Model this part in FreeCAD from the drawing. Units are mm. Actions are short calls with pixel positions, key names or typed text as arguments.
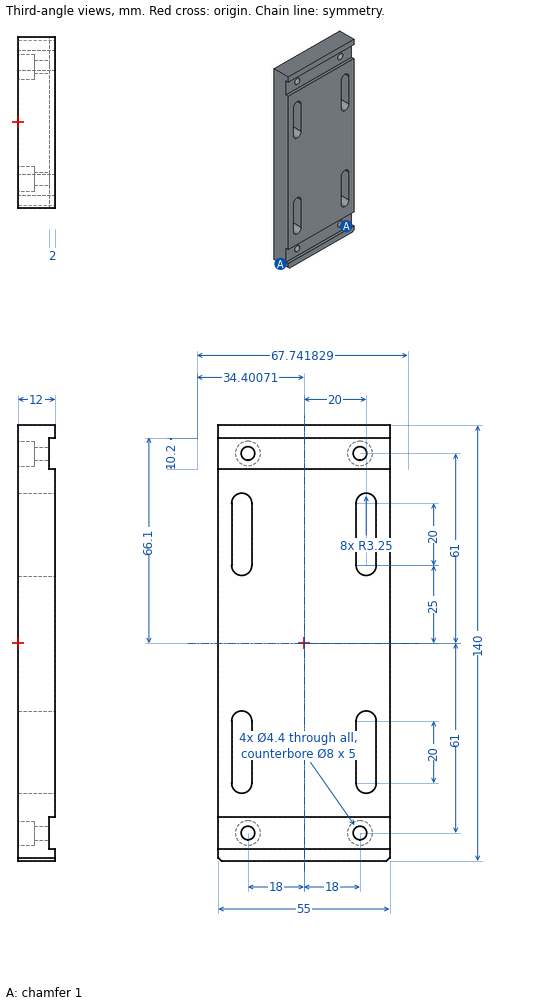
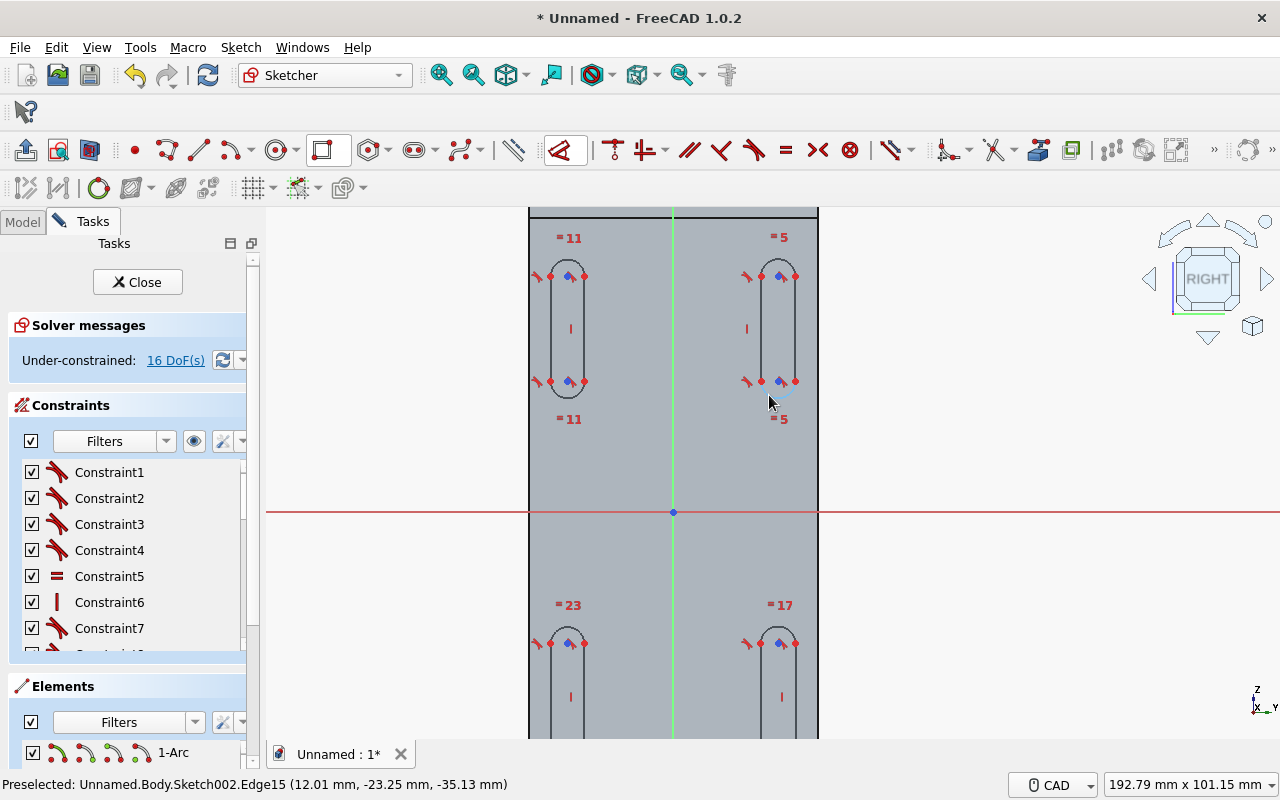
click(768, 395)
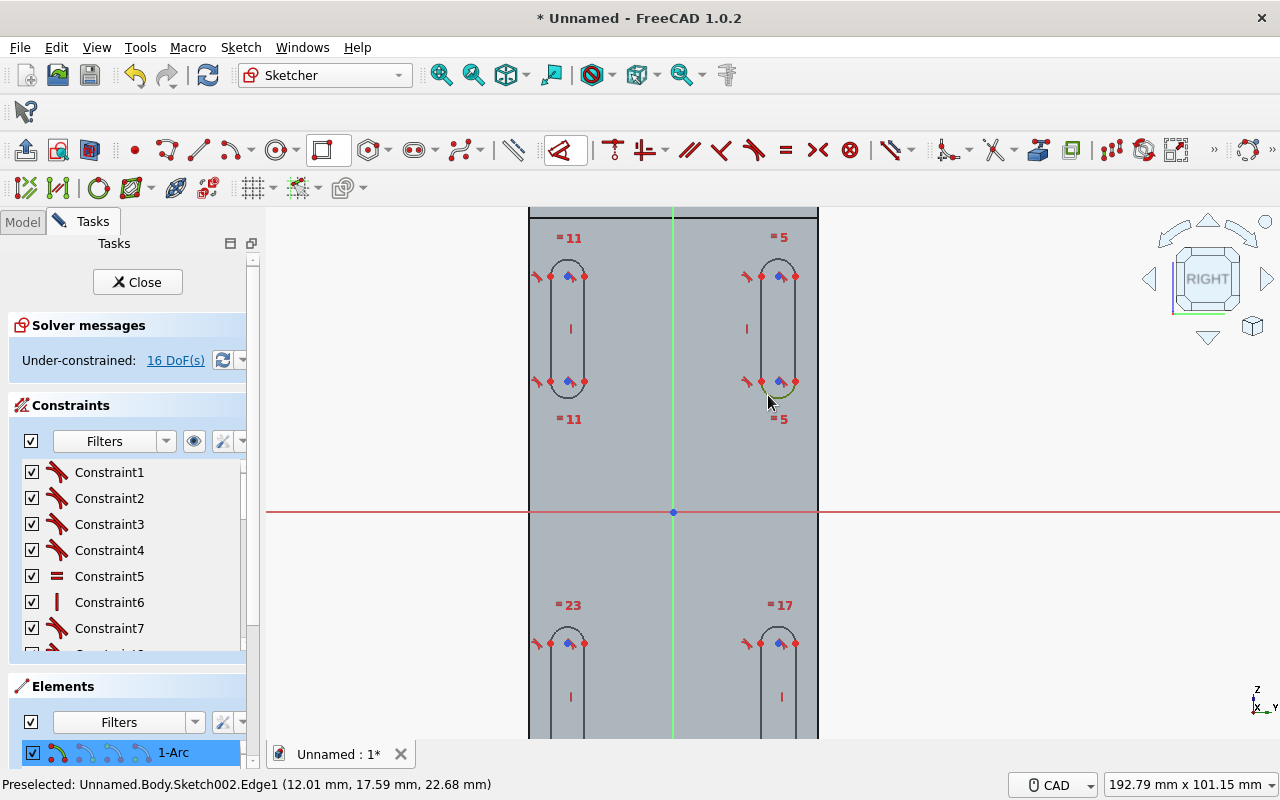
click(558, 395)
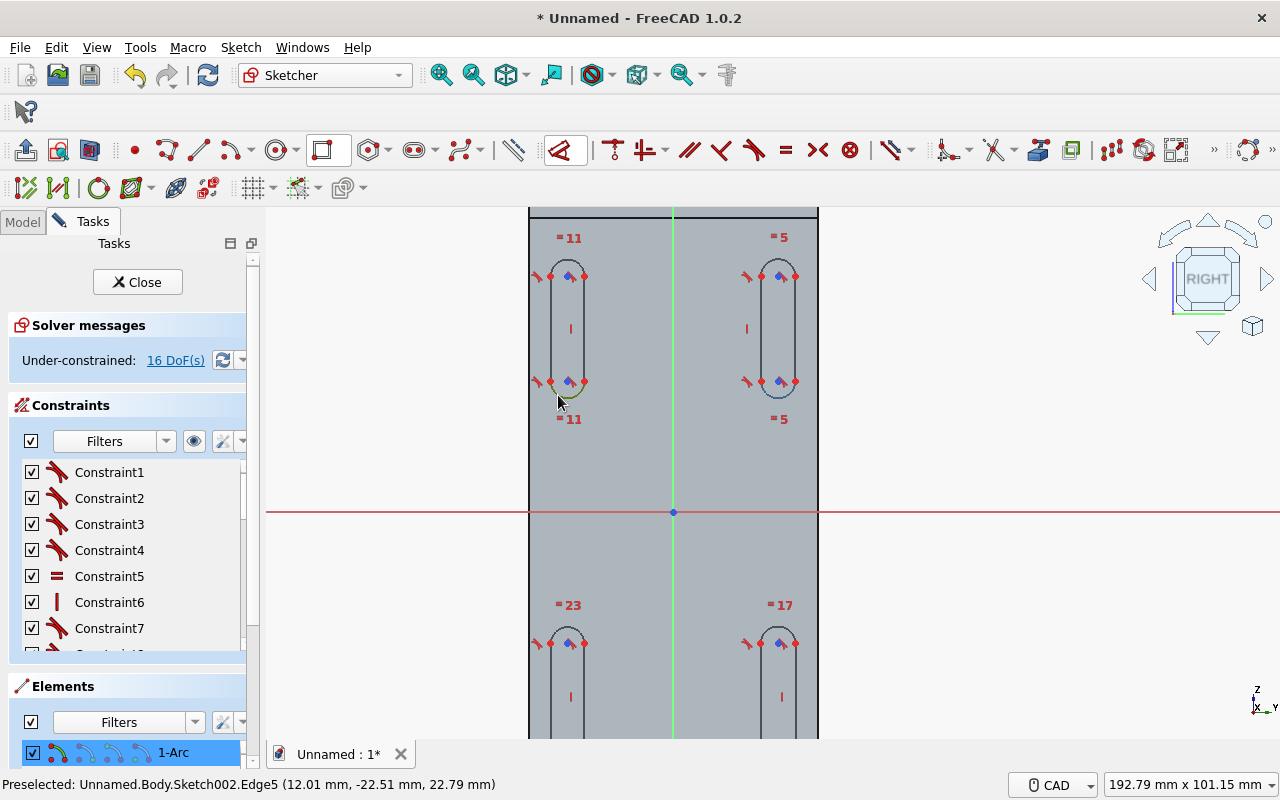
scroll(768, 393, down, 2)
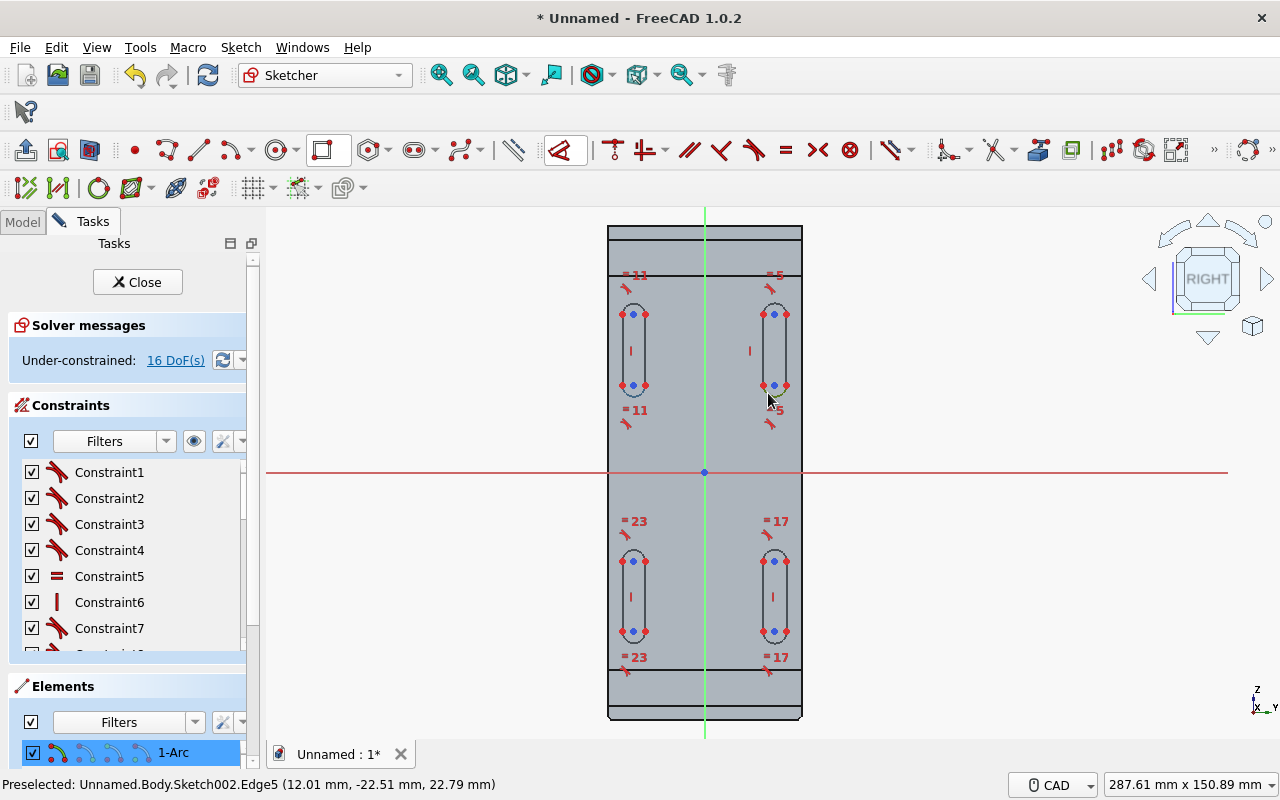
scroll(768, 641, up, 2)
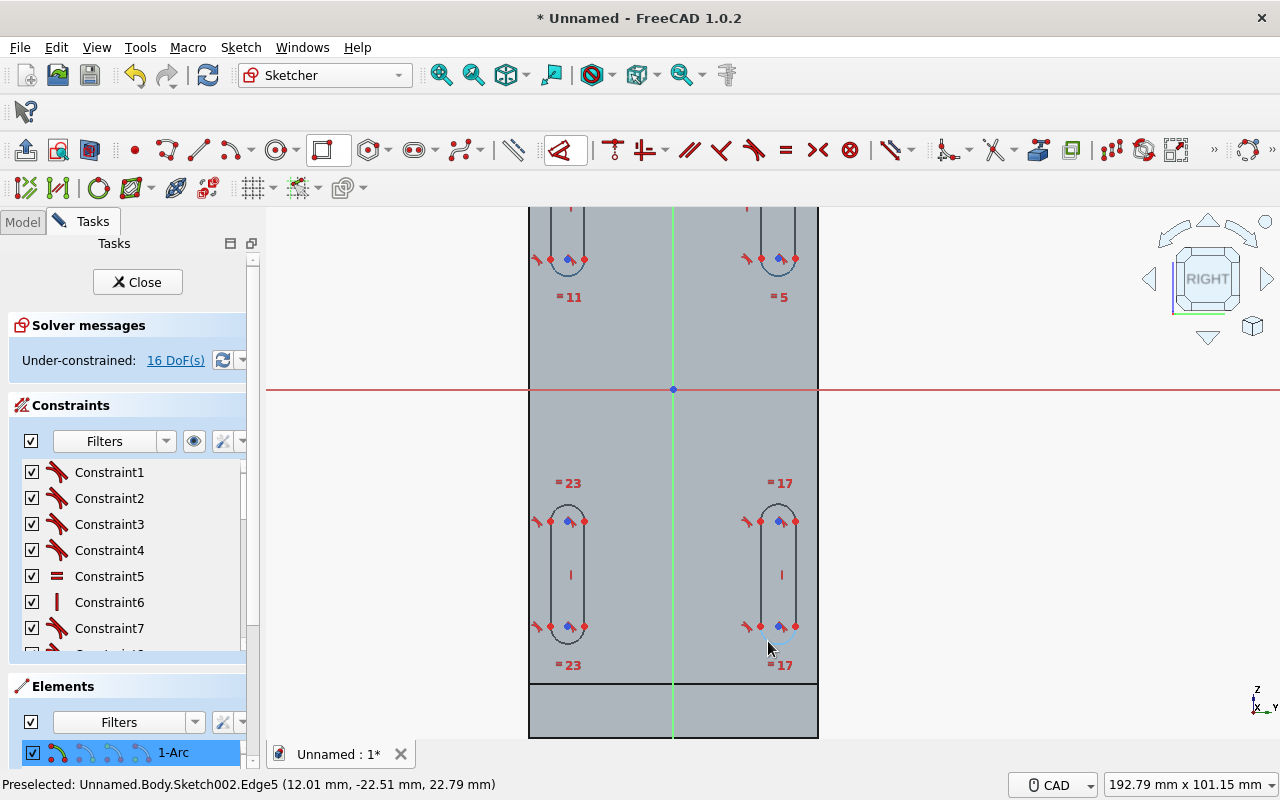
click(768, 641)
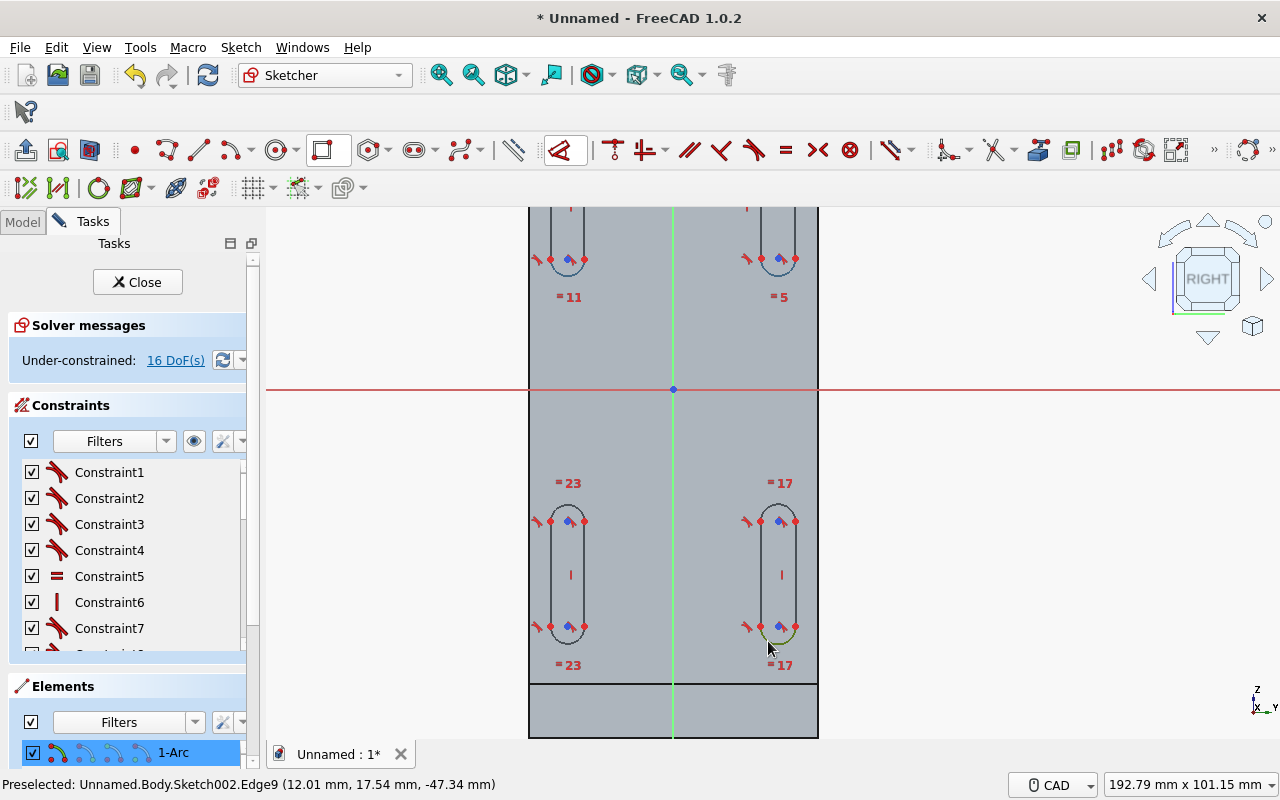
click(558, 641)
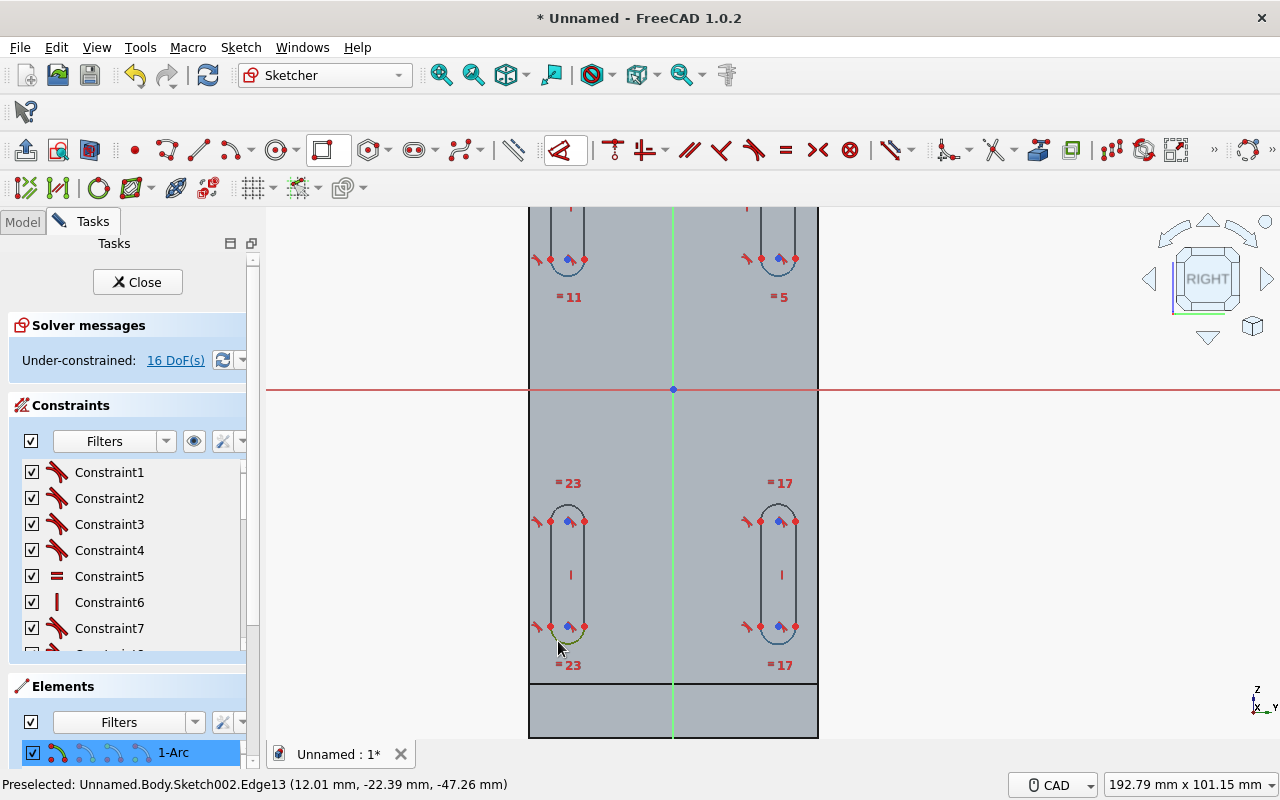
click(786, 150)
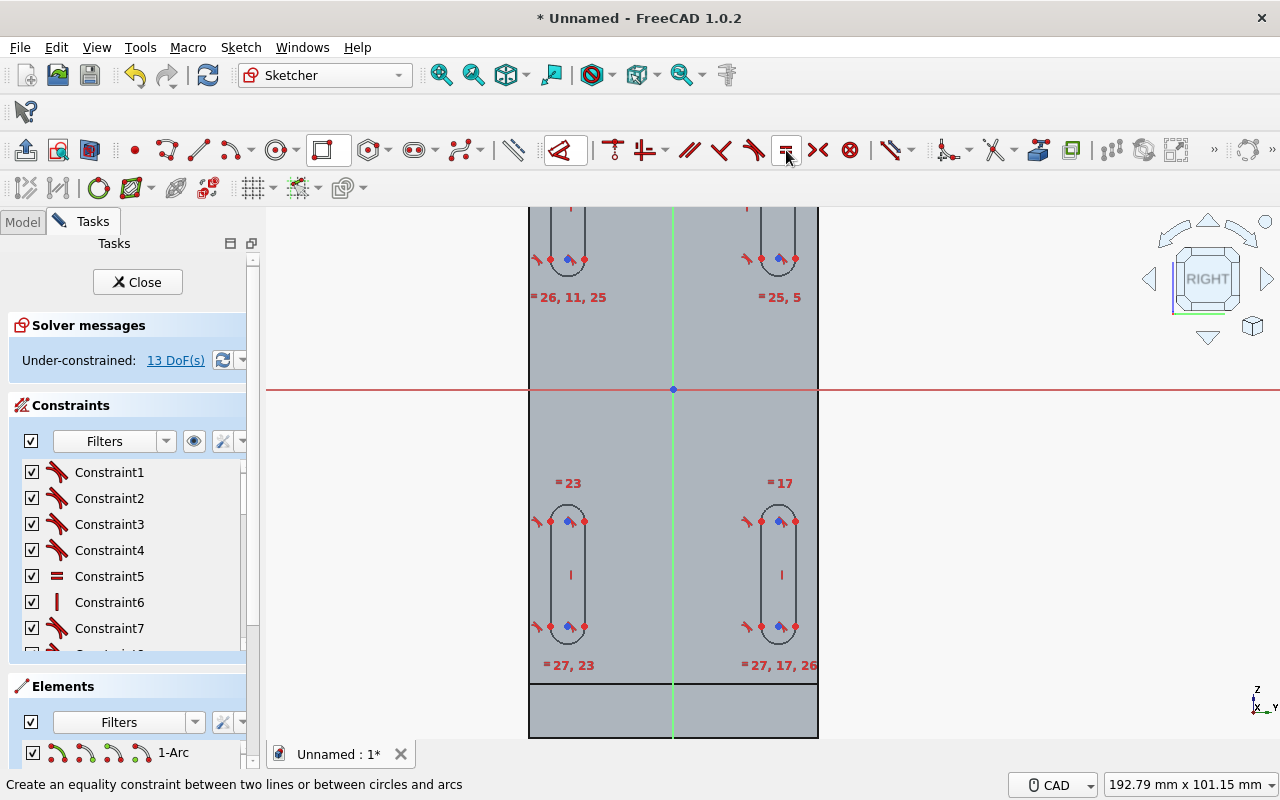
click(778, 259)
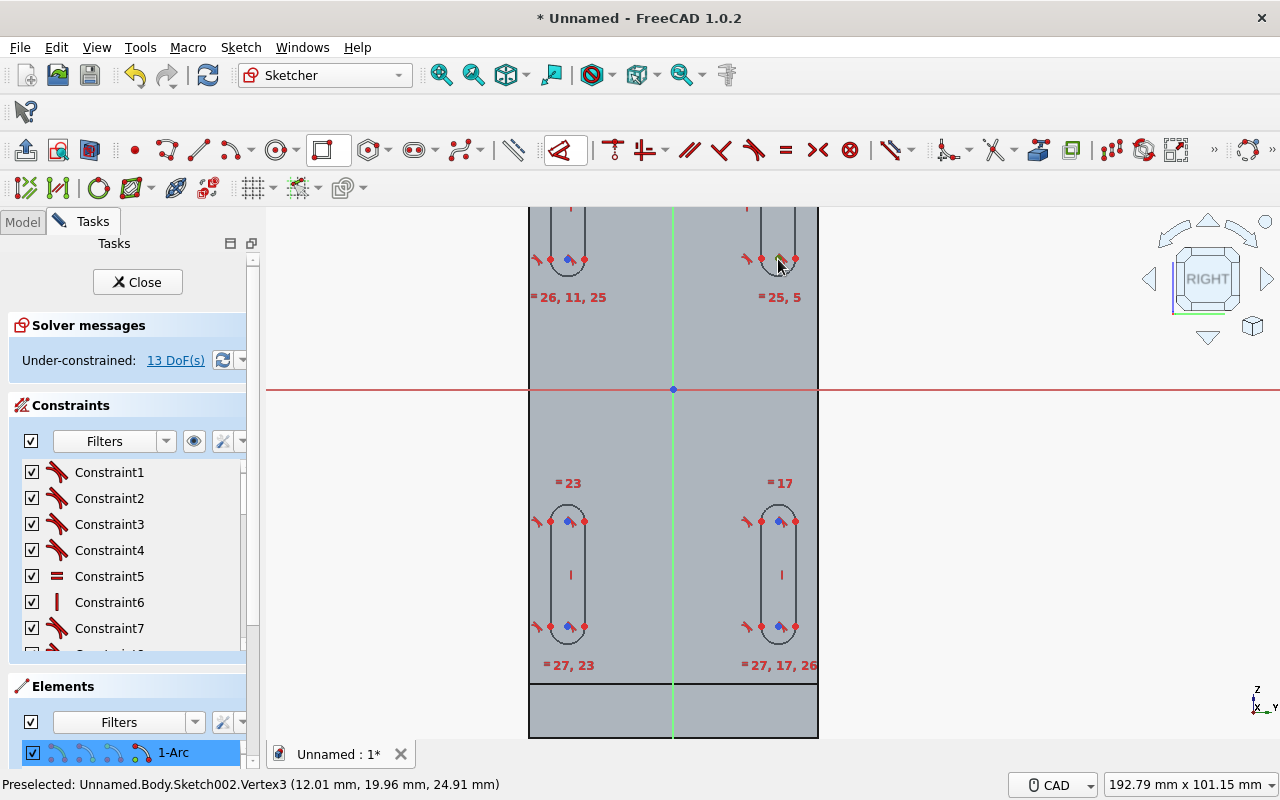
click(568, 259)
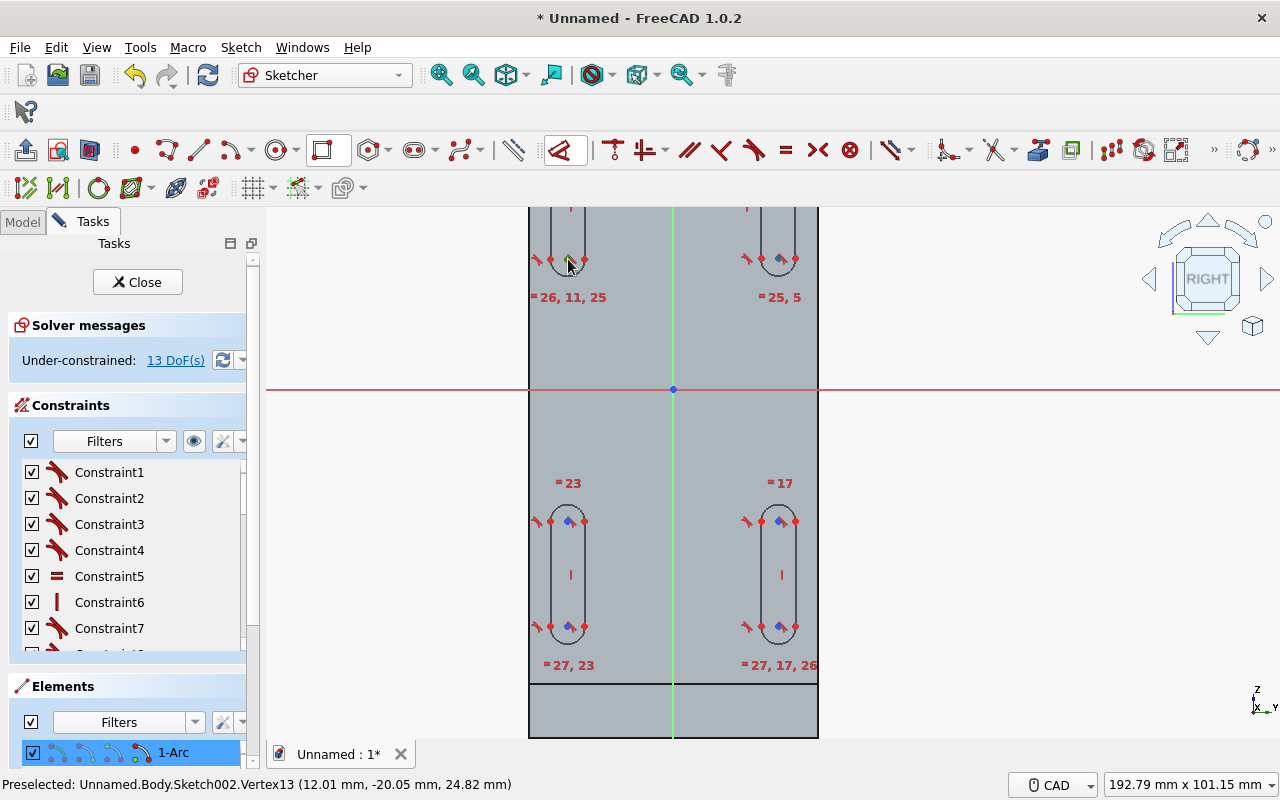
click(673, 677)